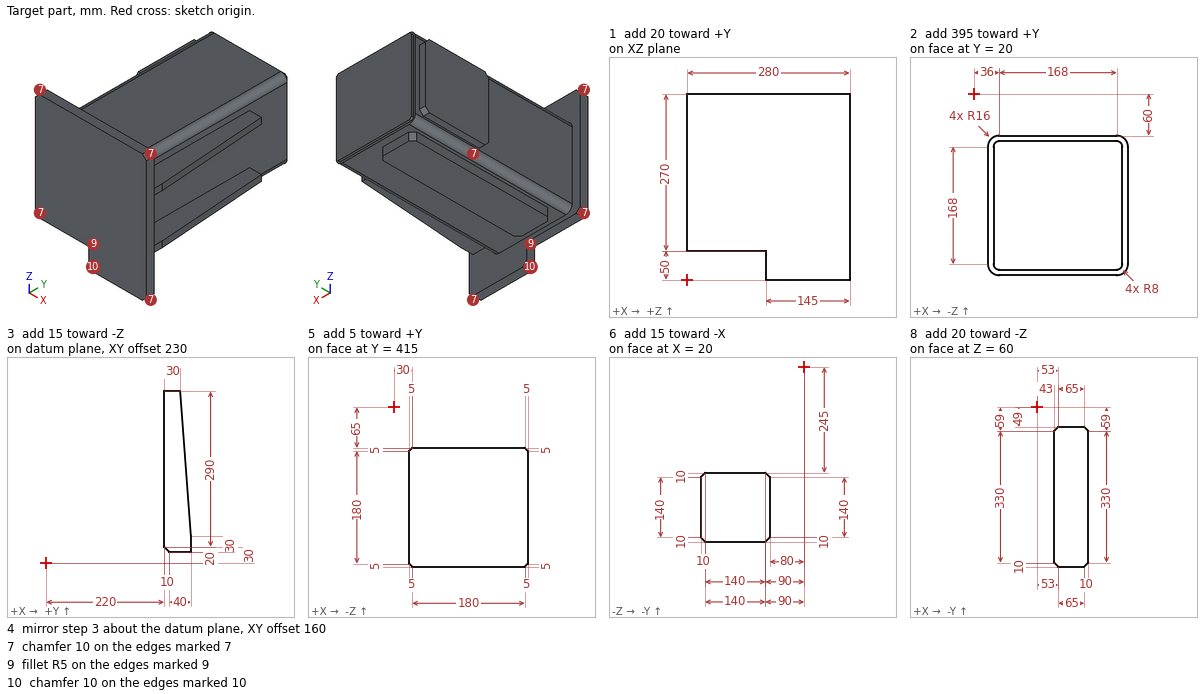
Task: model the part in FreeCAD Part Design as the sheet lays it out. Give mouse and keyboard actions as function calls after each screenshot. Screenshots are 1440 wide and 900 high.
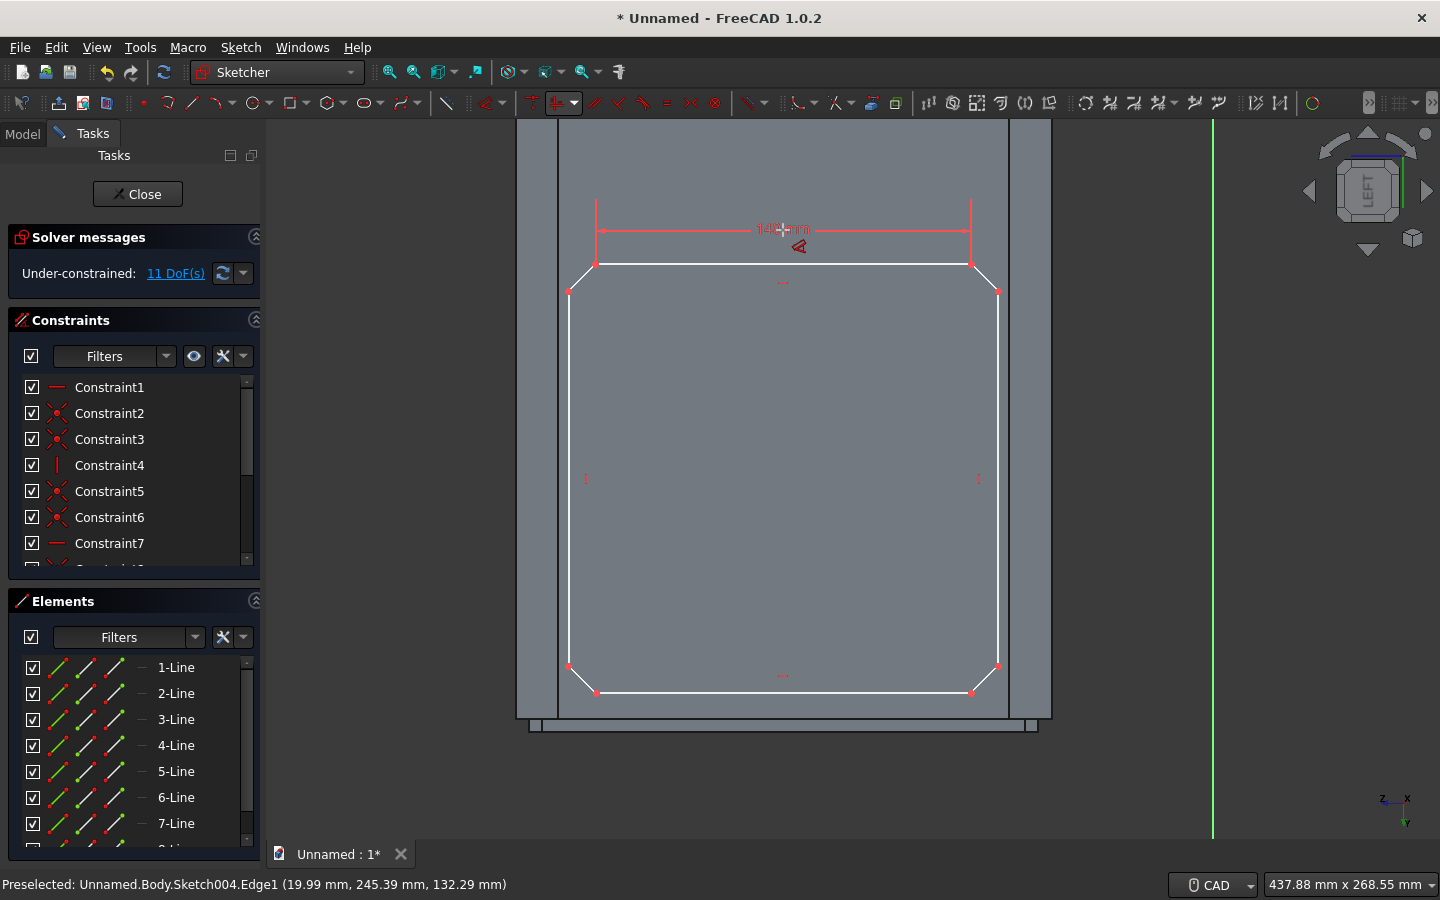
click(569, 403)
click(535, 478)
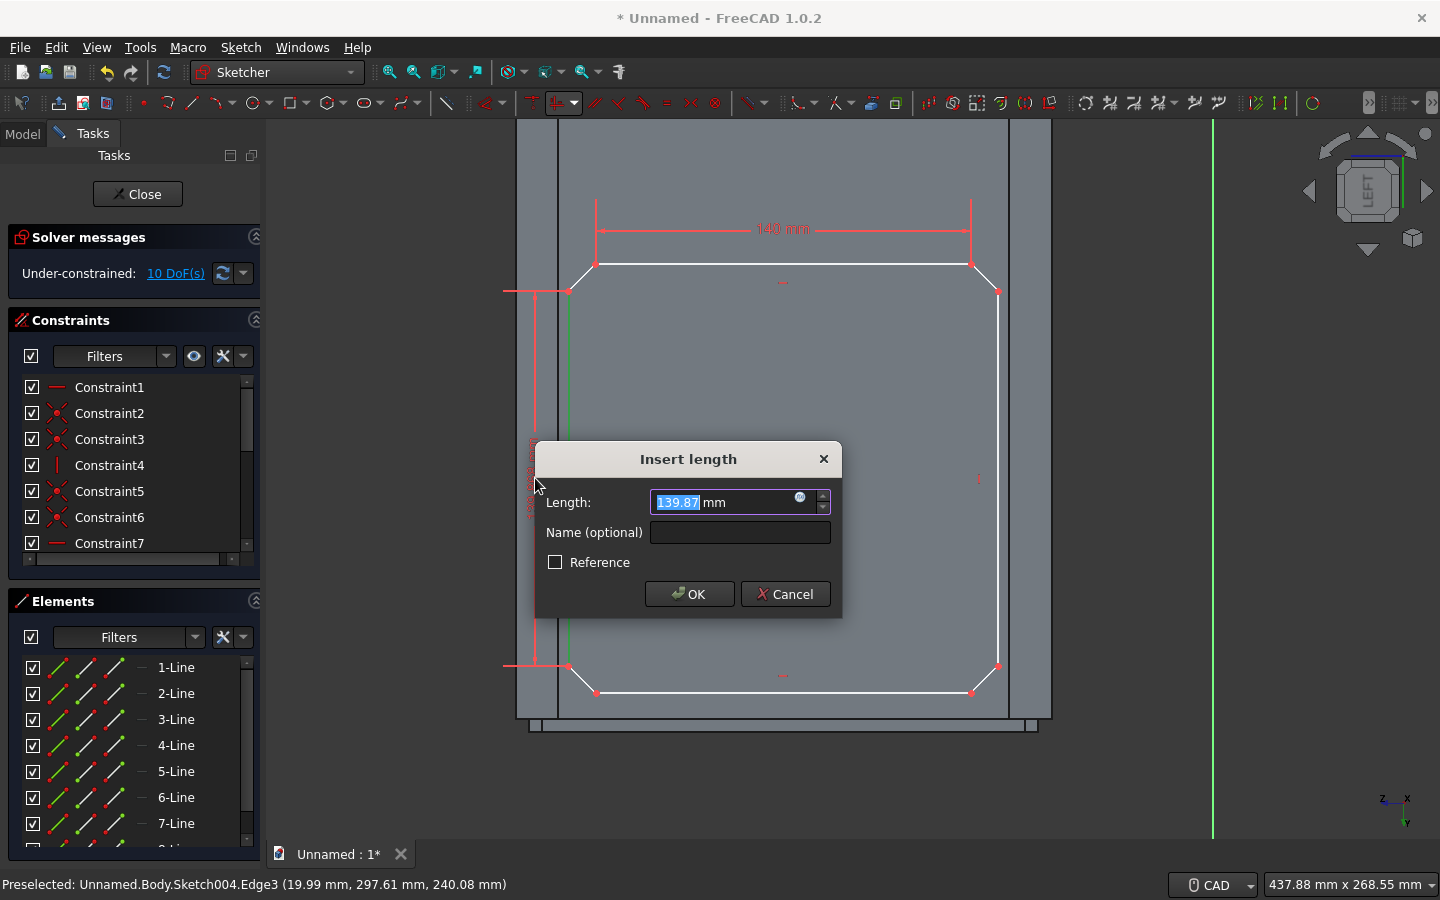
text(140)
key(Return)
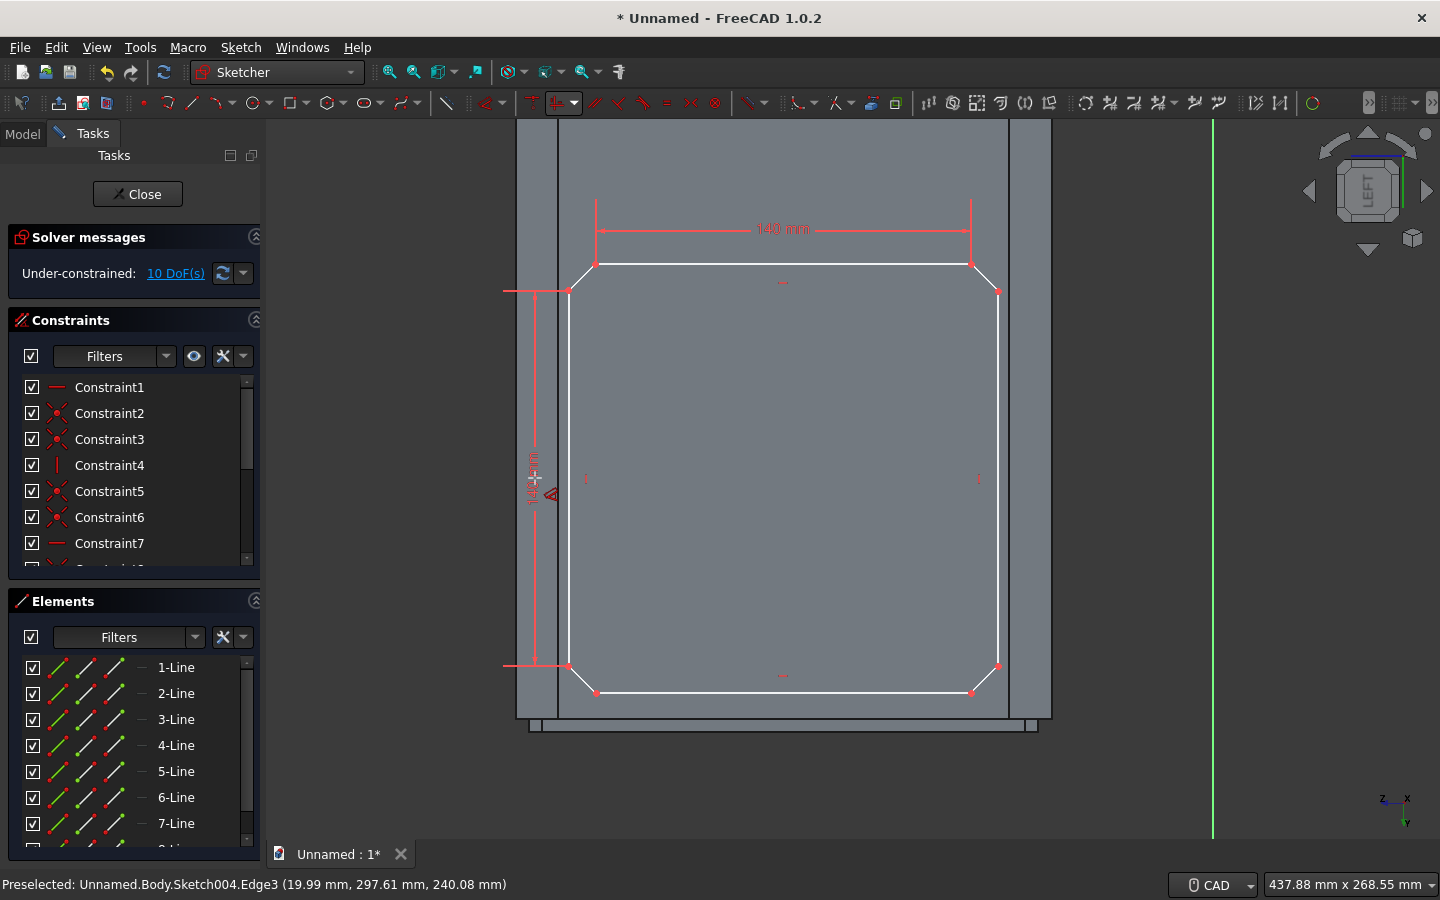
click(709, 693)
click(783, 727)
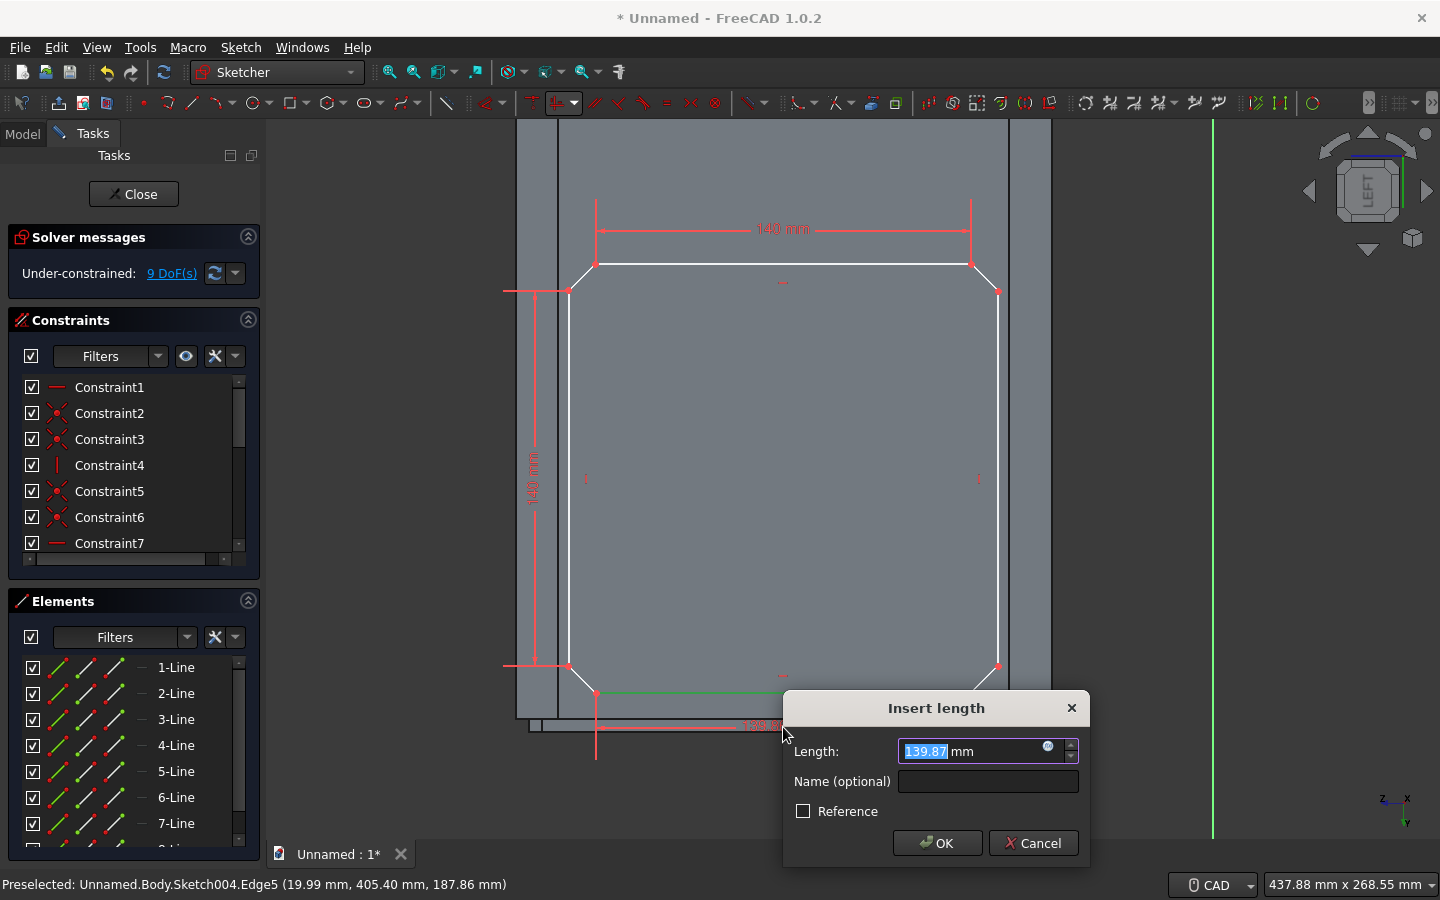
text(140)
key(Return)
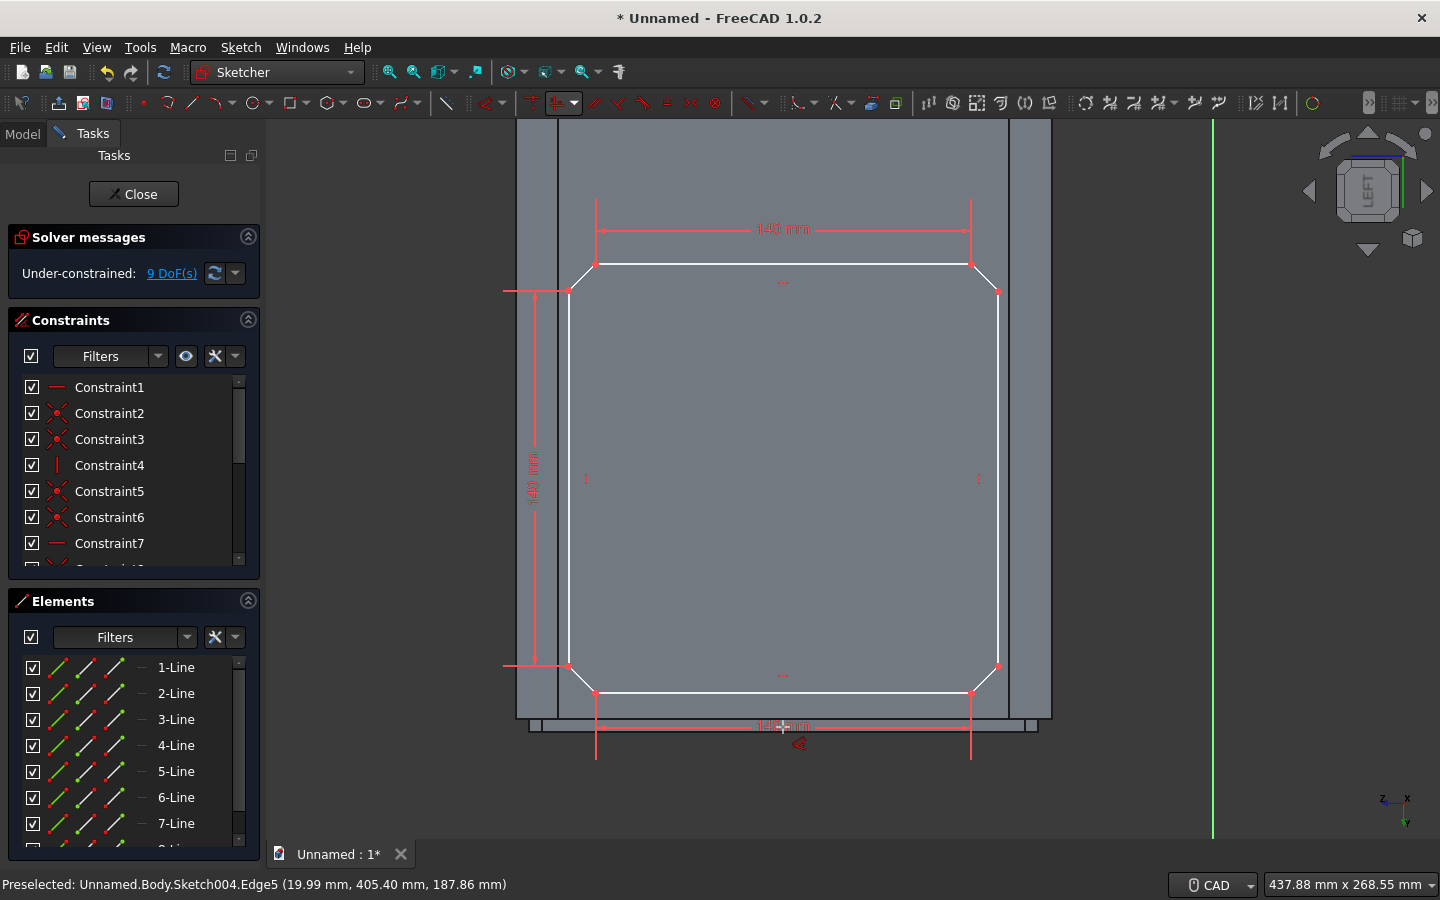
click(998, 553)
click(1032, 478)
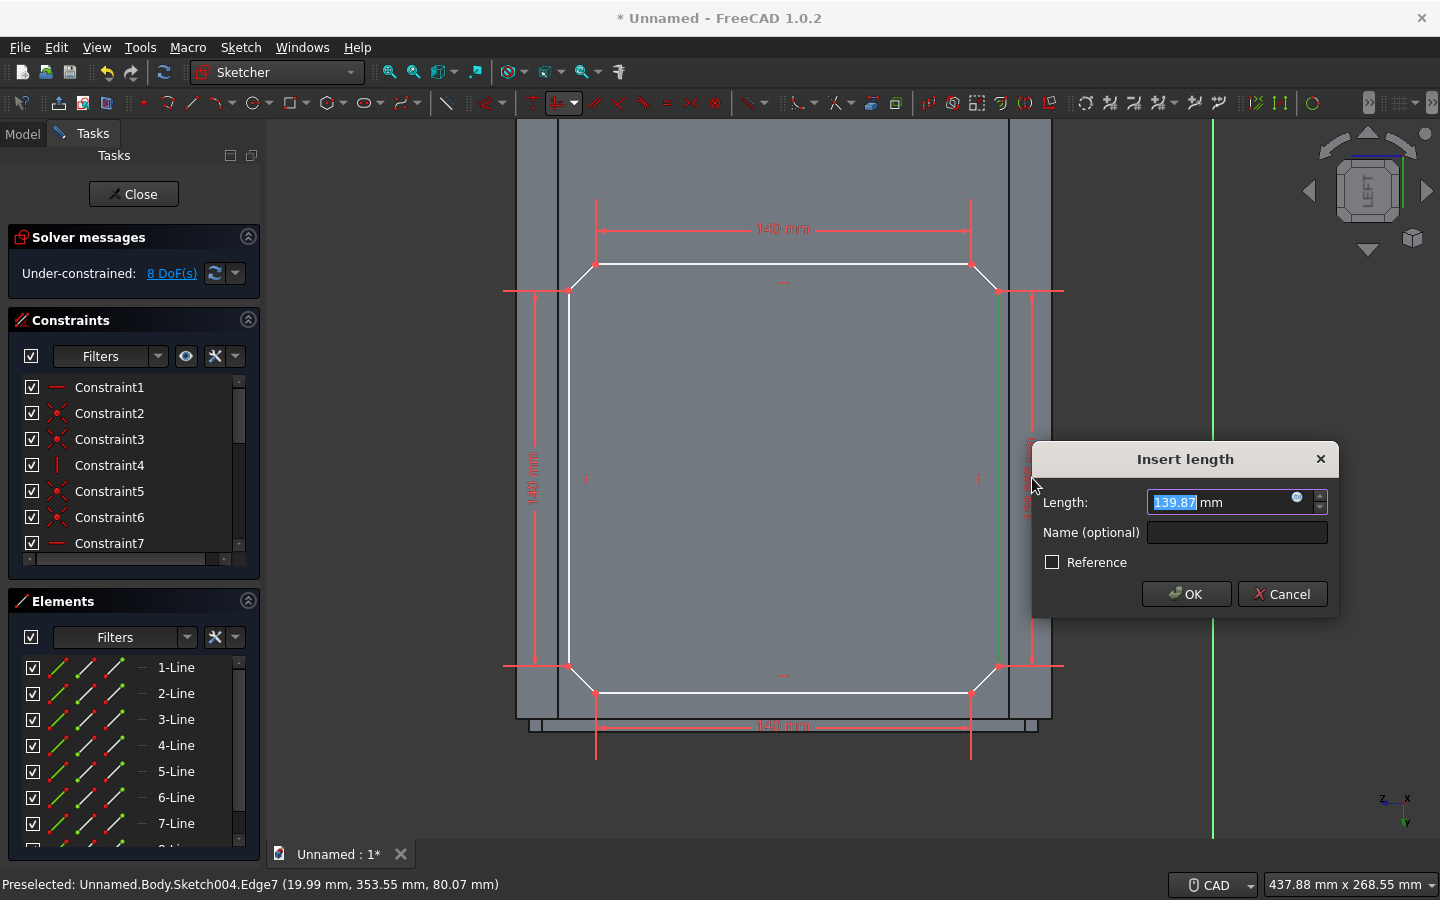
text(140)
key(Return)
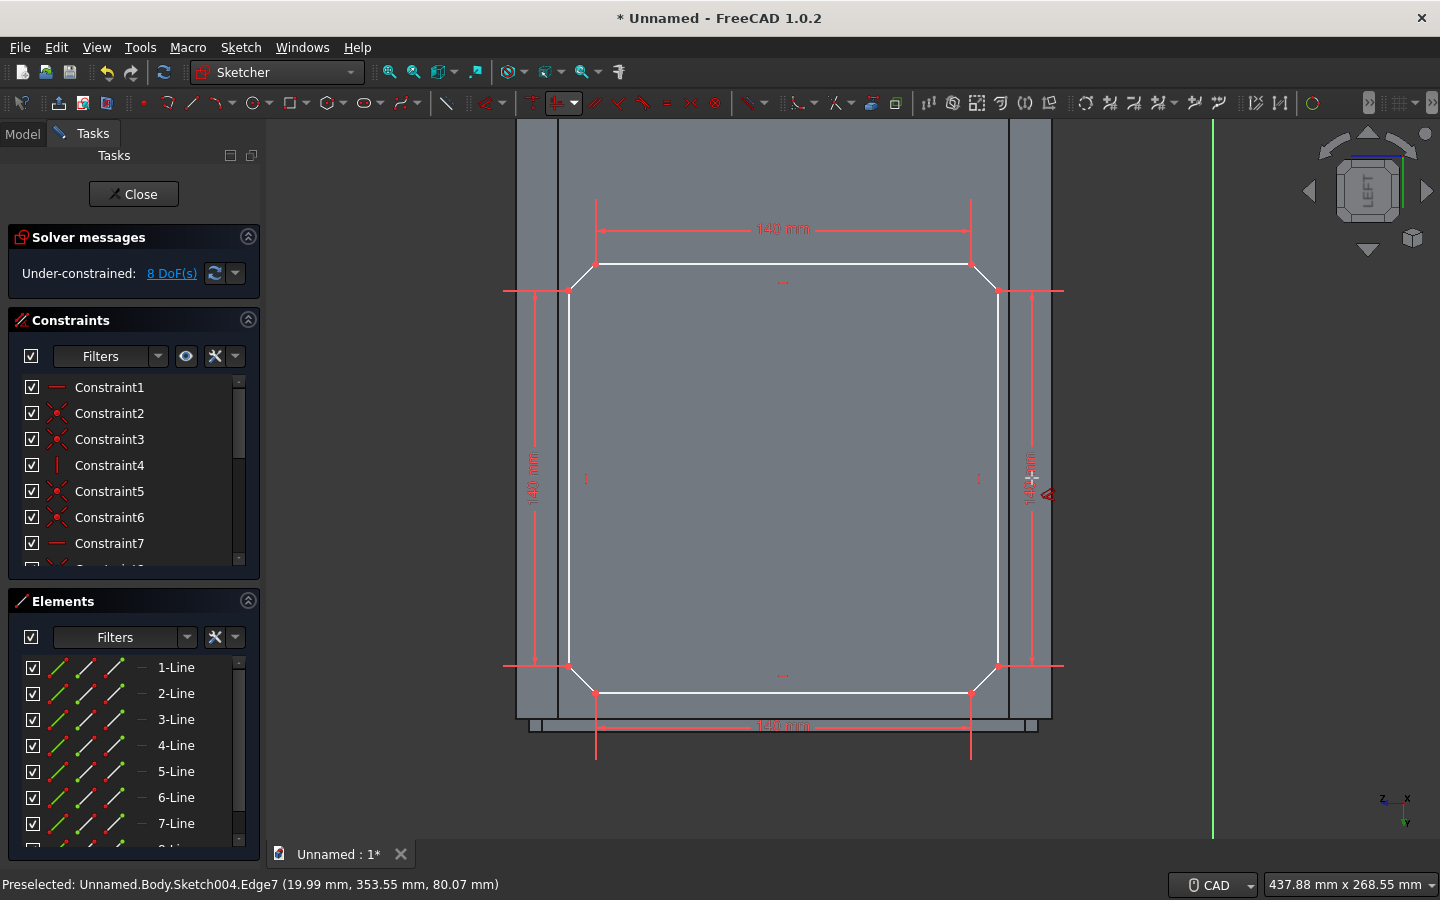
click(971, 264)
click(1092, 298)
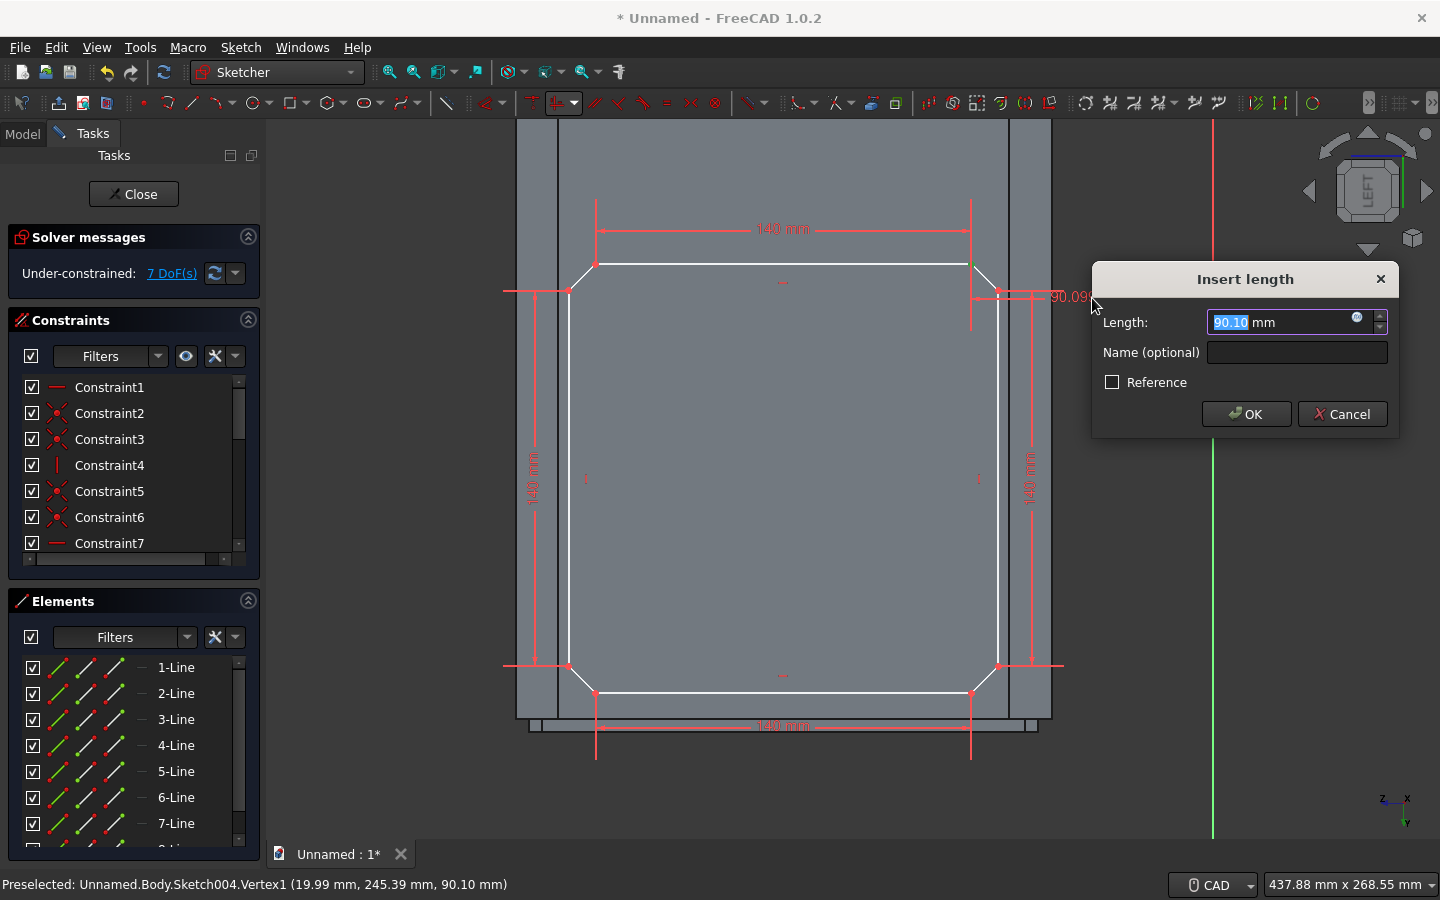
text(90)
key(Return)